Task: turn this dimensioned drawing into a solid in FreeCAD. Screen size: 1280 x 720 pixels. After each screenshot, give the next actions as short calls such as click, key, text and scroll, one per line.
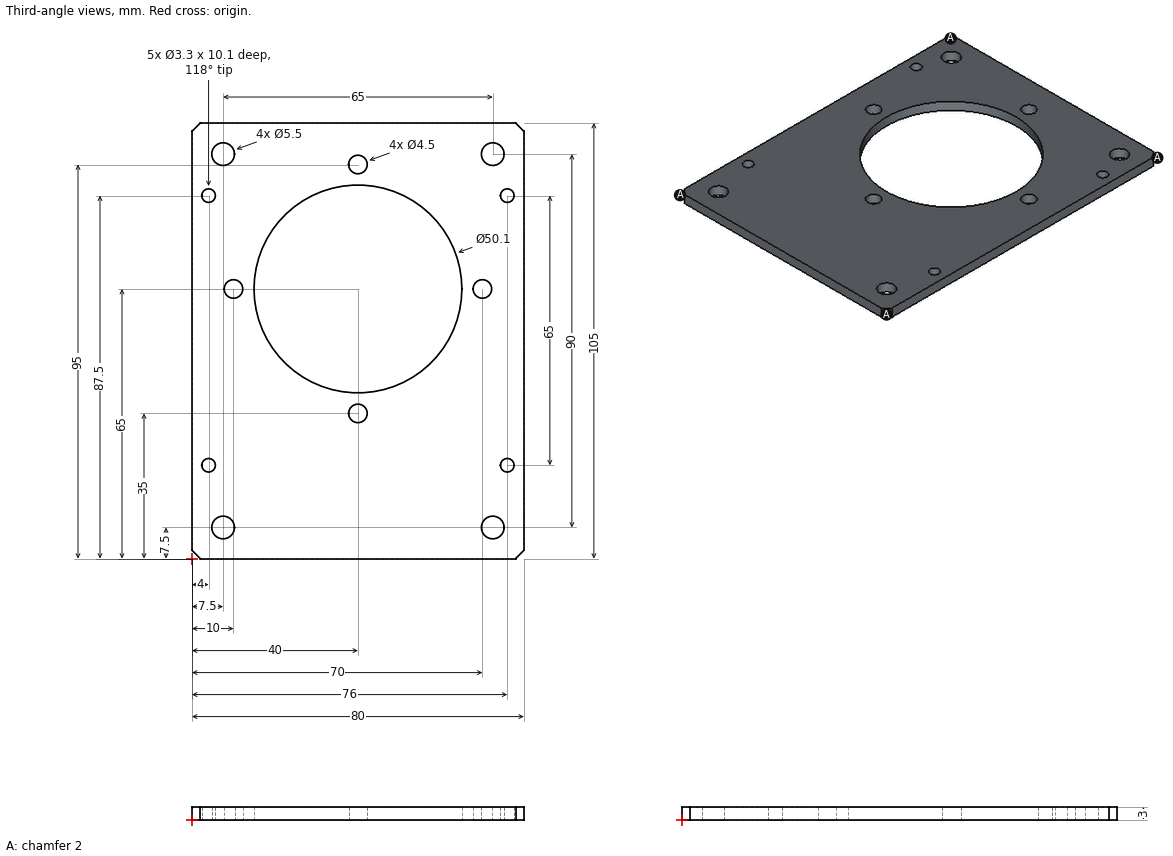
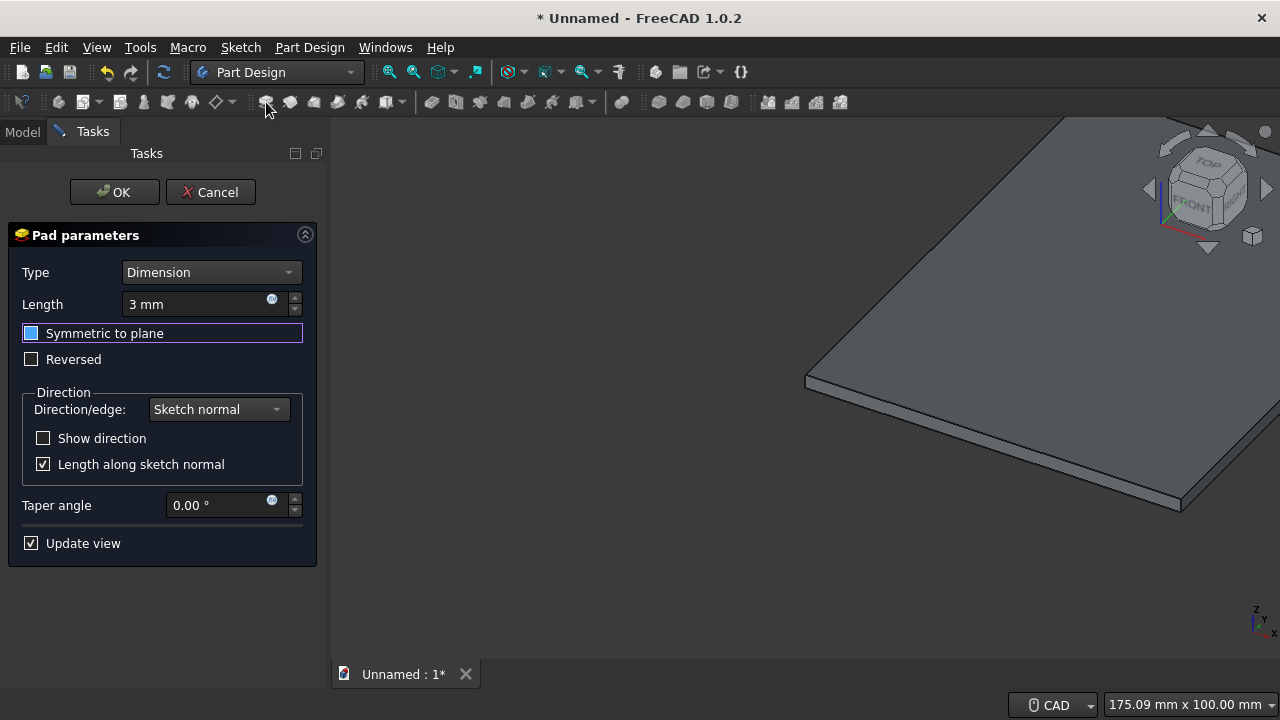
click(115, 192)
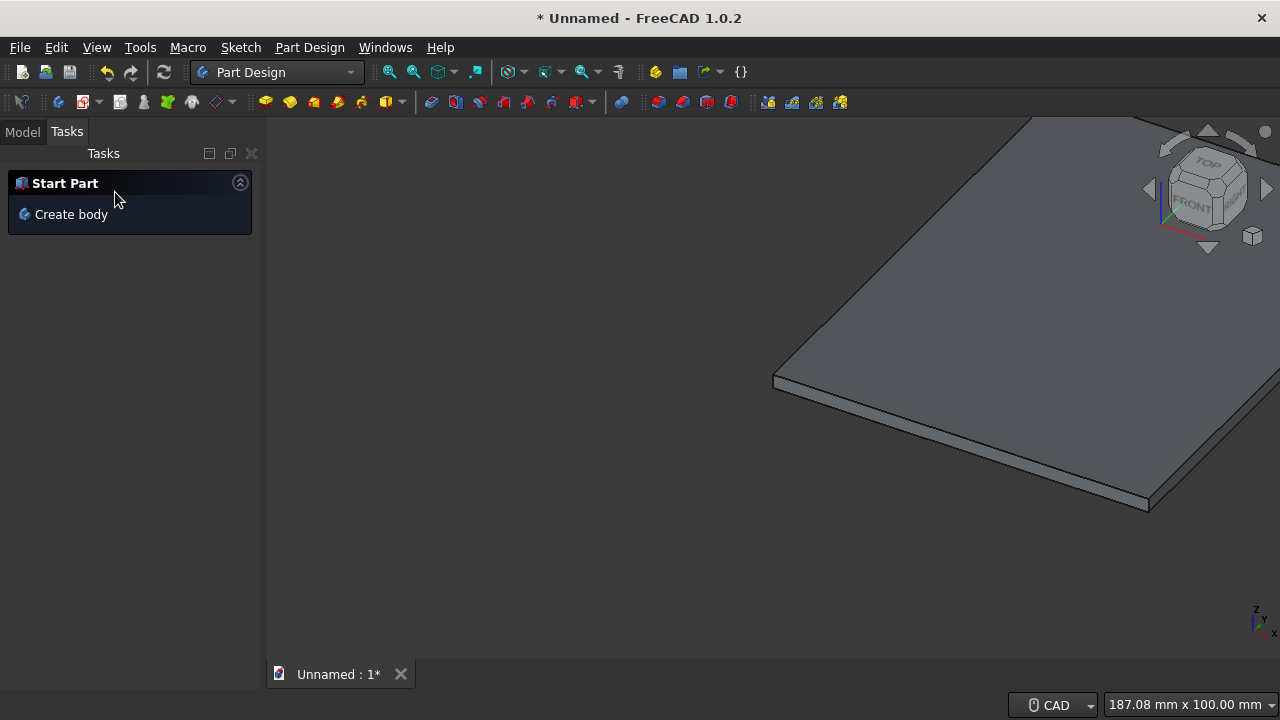
key(v)
key(f)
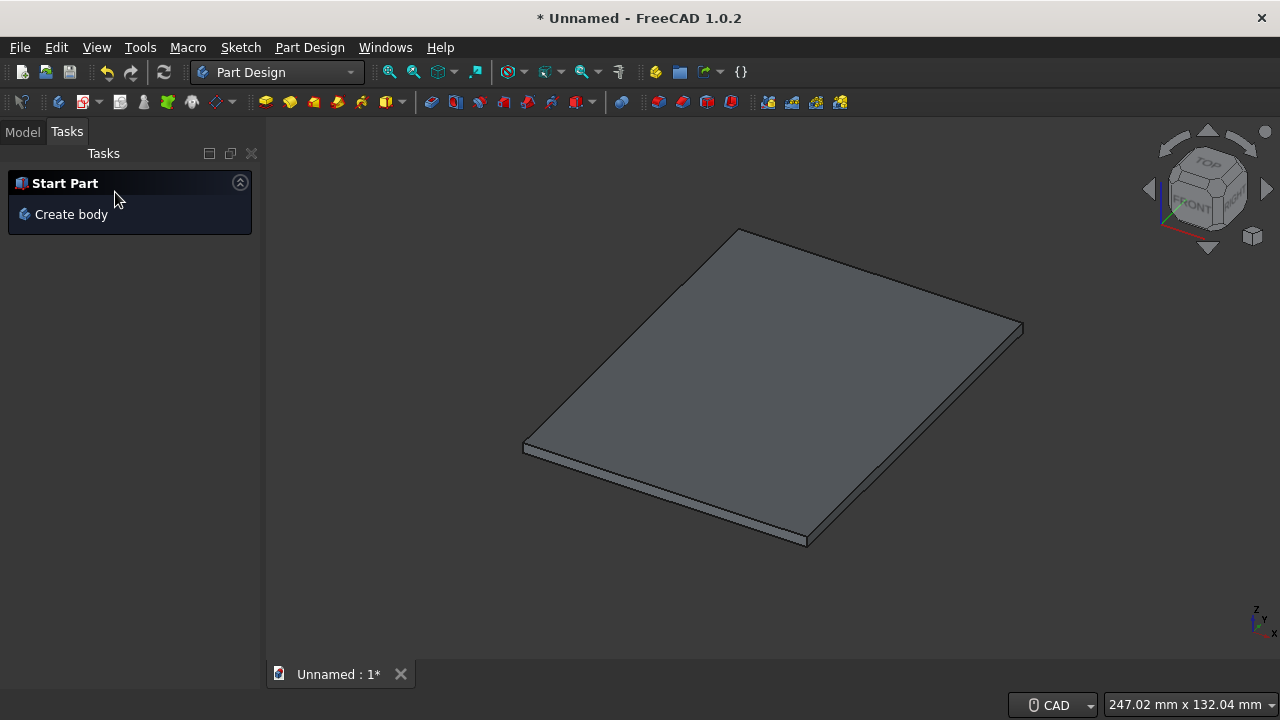
click(773, 382)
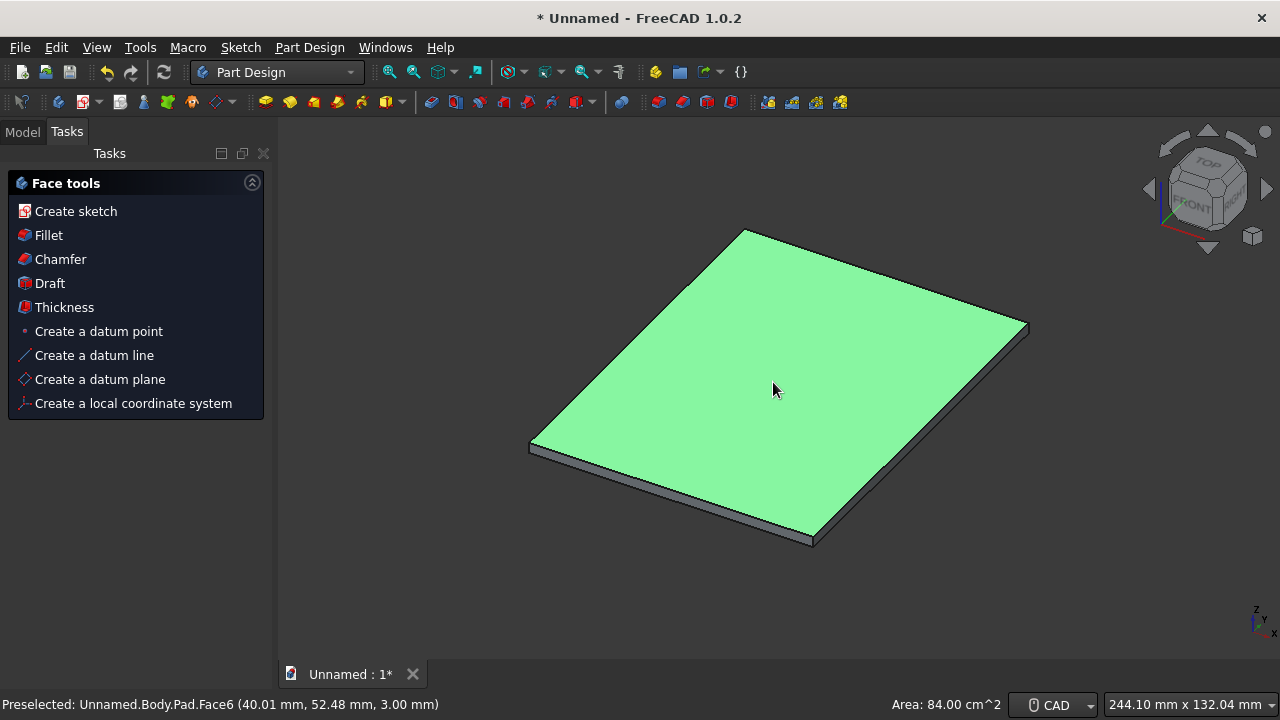
click(84, 102)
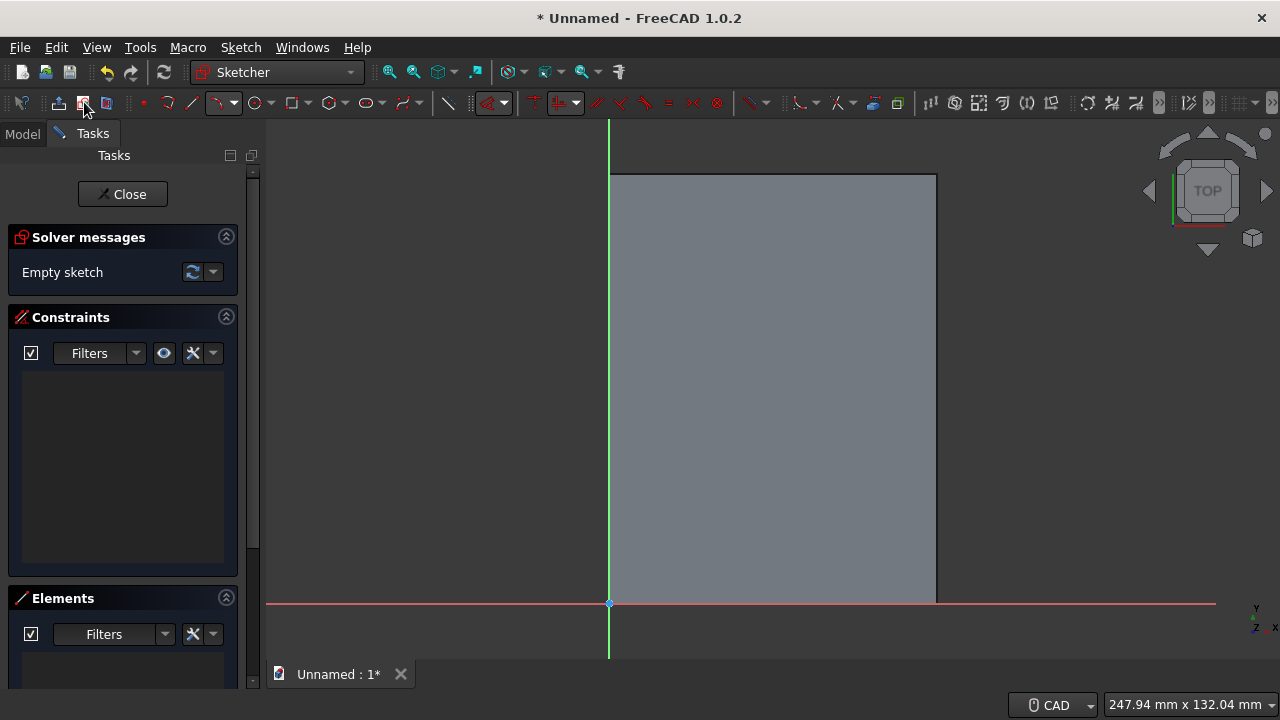
click(256, 104)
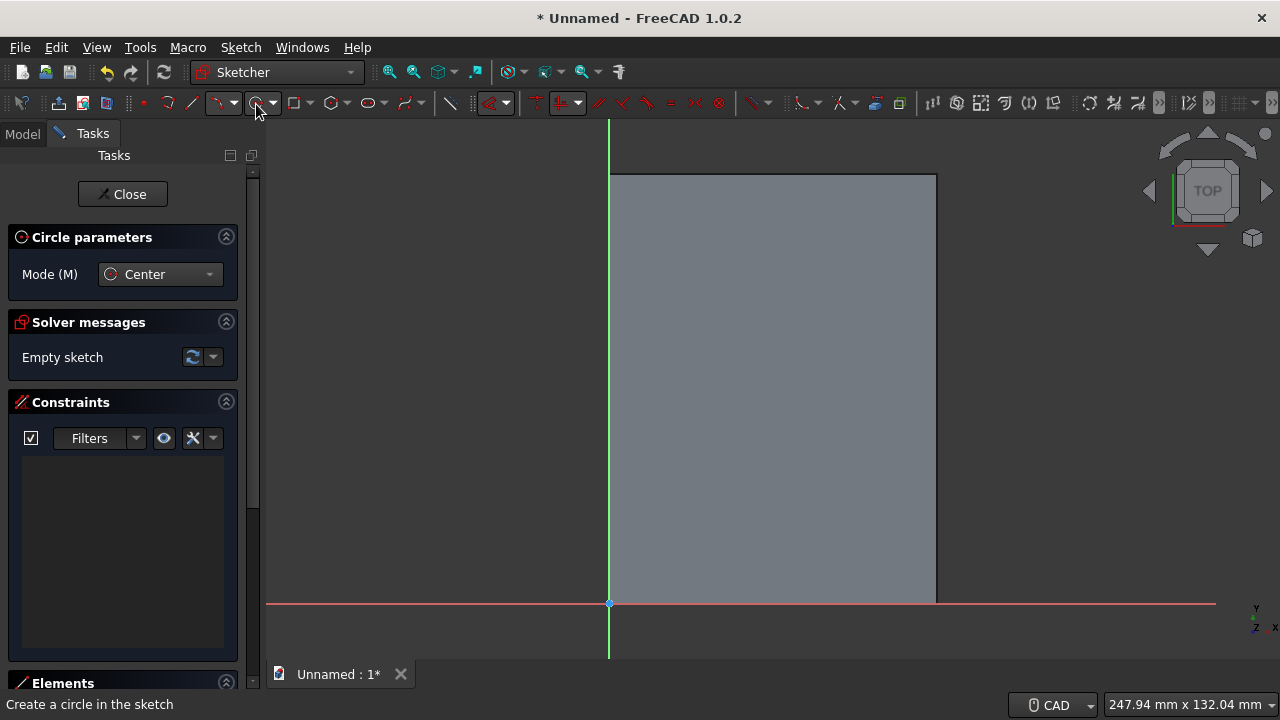
scroll(640, 205, up, 4)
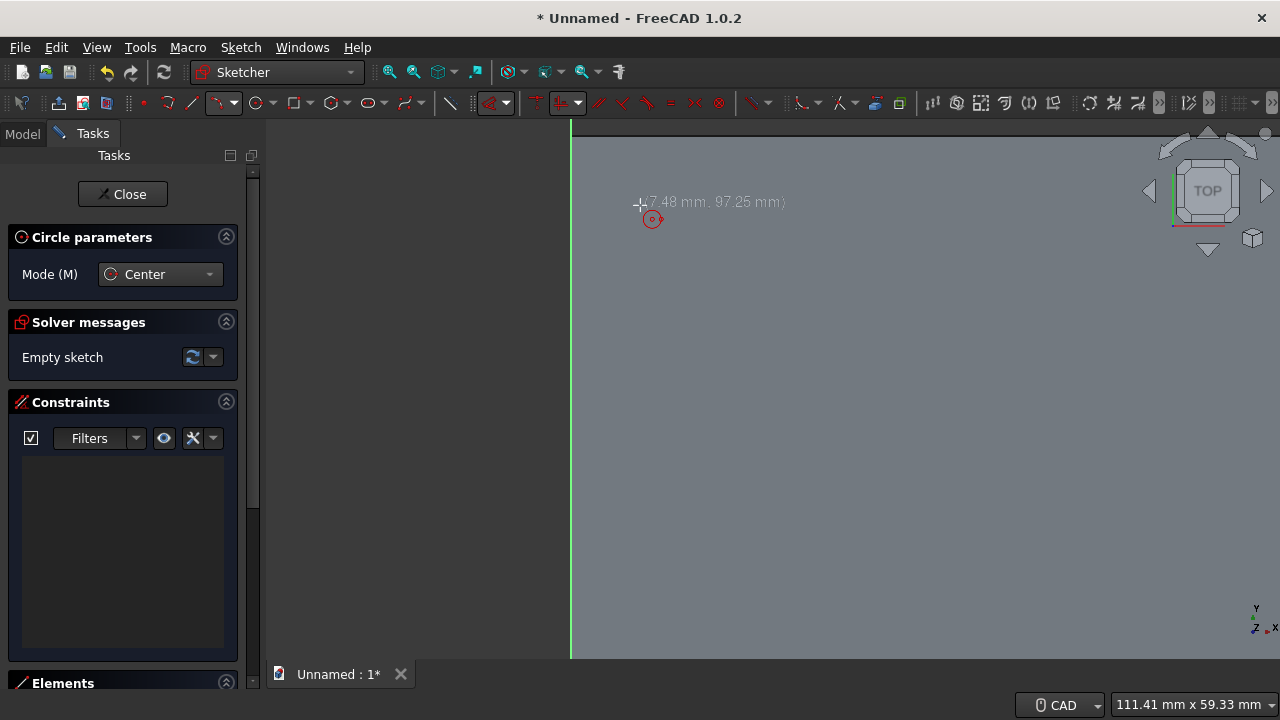
click(640, 205)
move(657, 187)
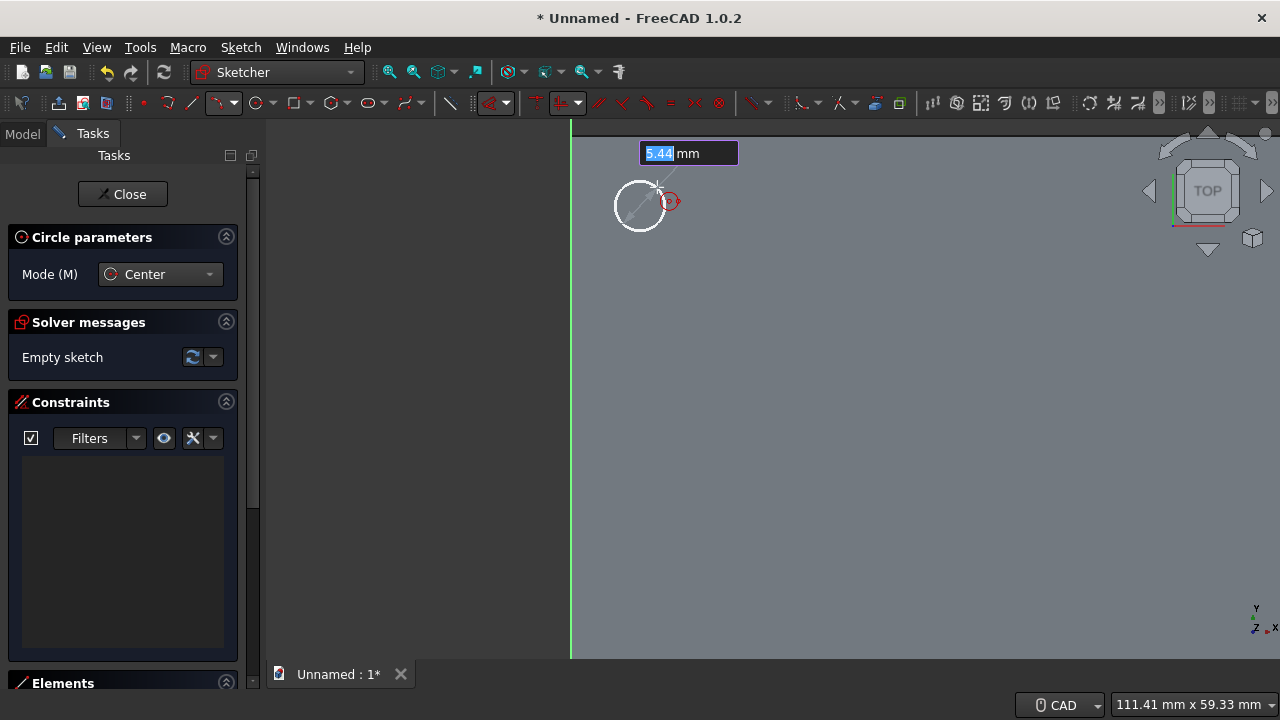
text(5.5)
key(Return)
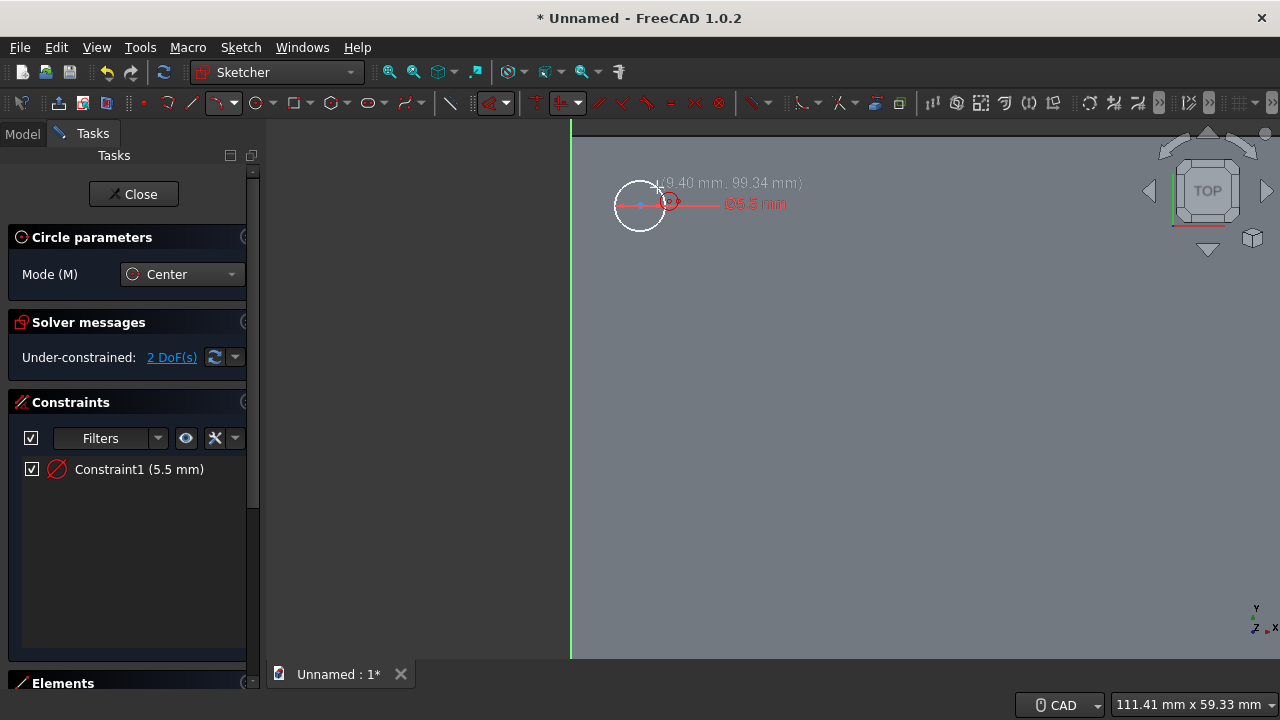
scroll(583, 245, down, 5)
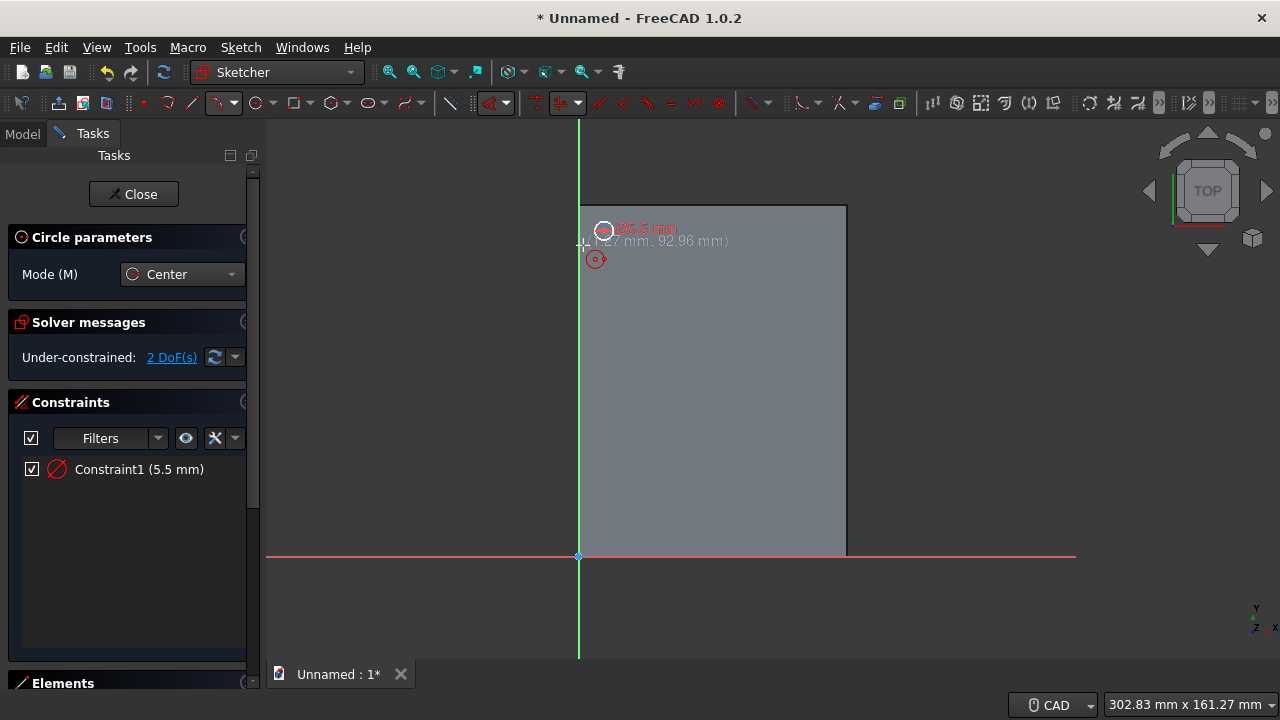
scroll(822, 230, up, 5)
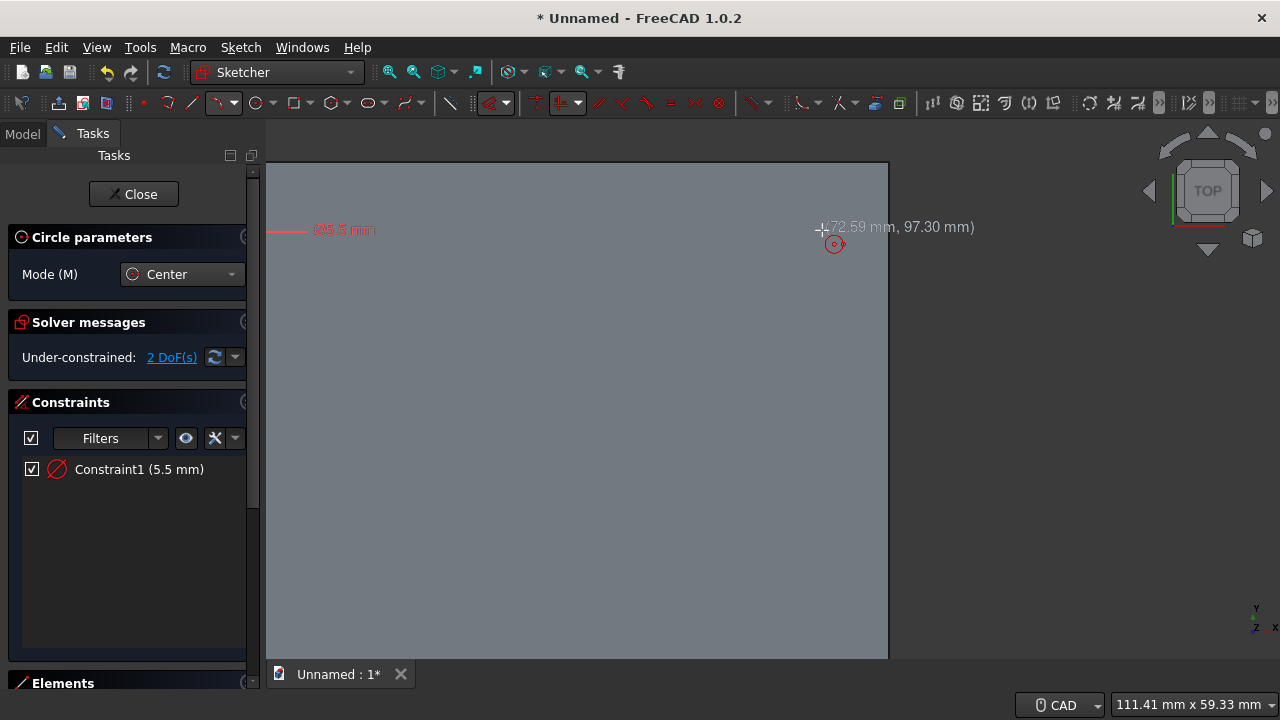
click(820, 231)
move(838, 213)